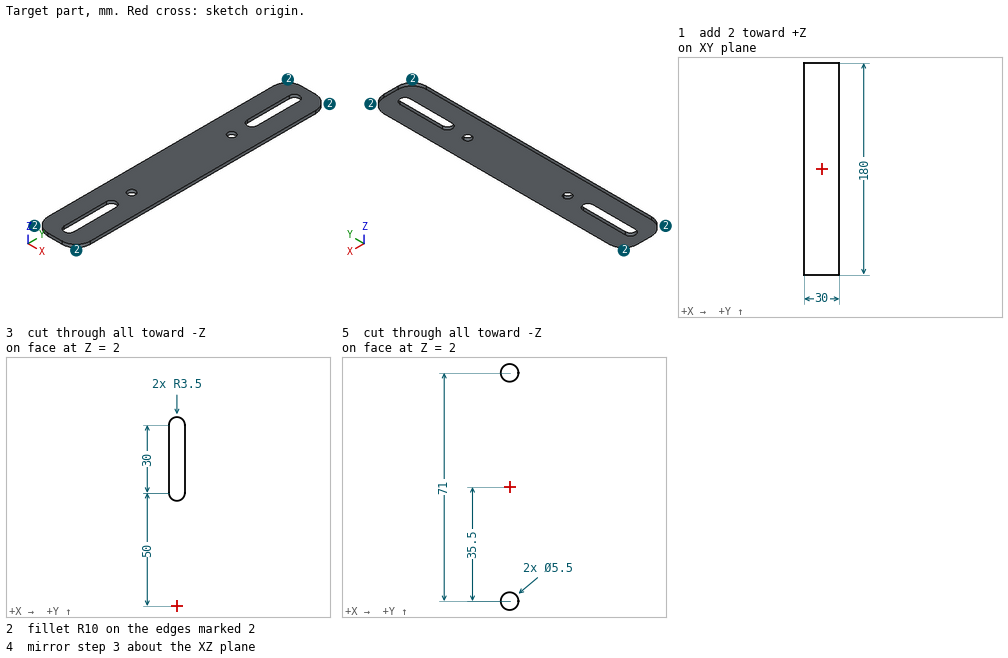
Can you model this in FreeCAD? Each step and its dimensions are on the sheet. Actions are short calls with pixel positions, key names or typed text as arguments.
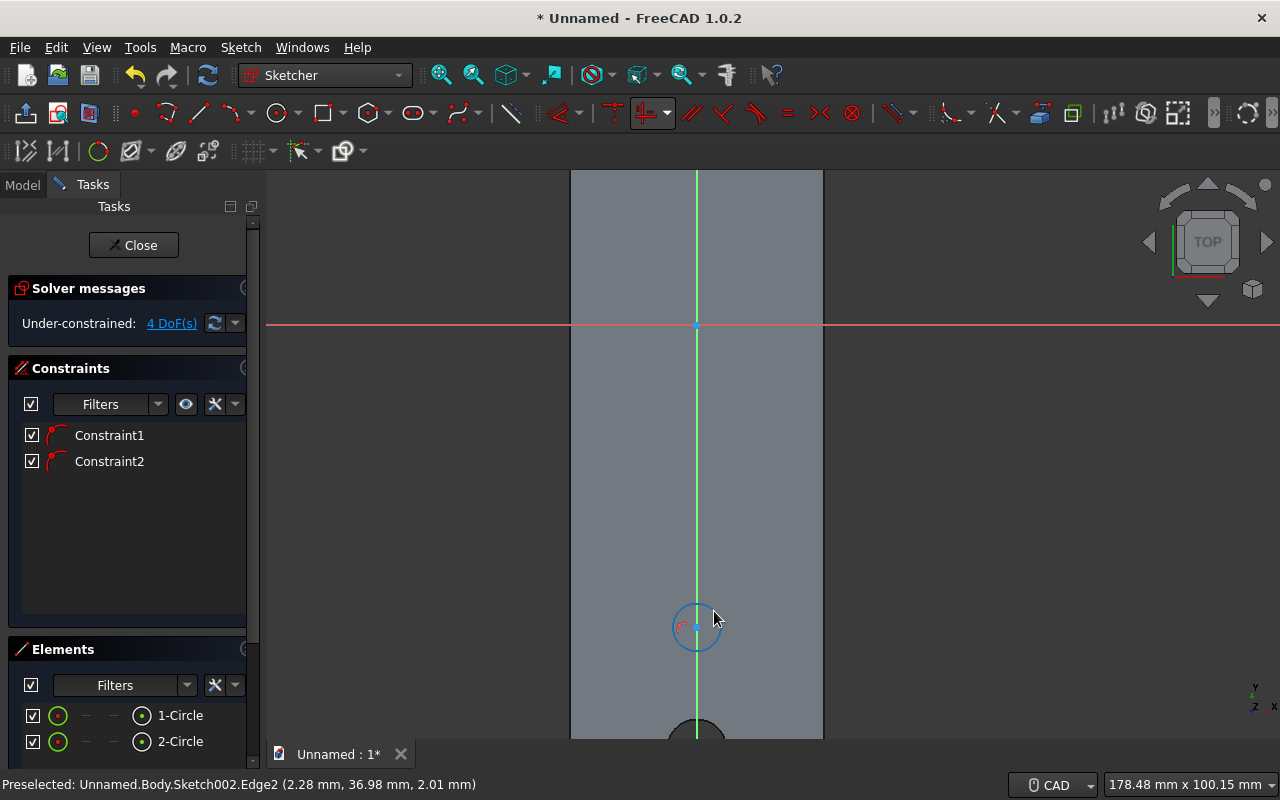
click(714, 610)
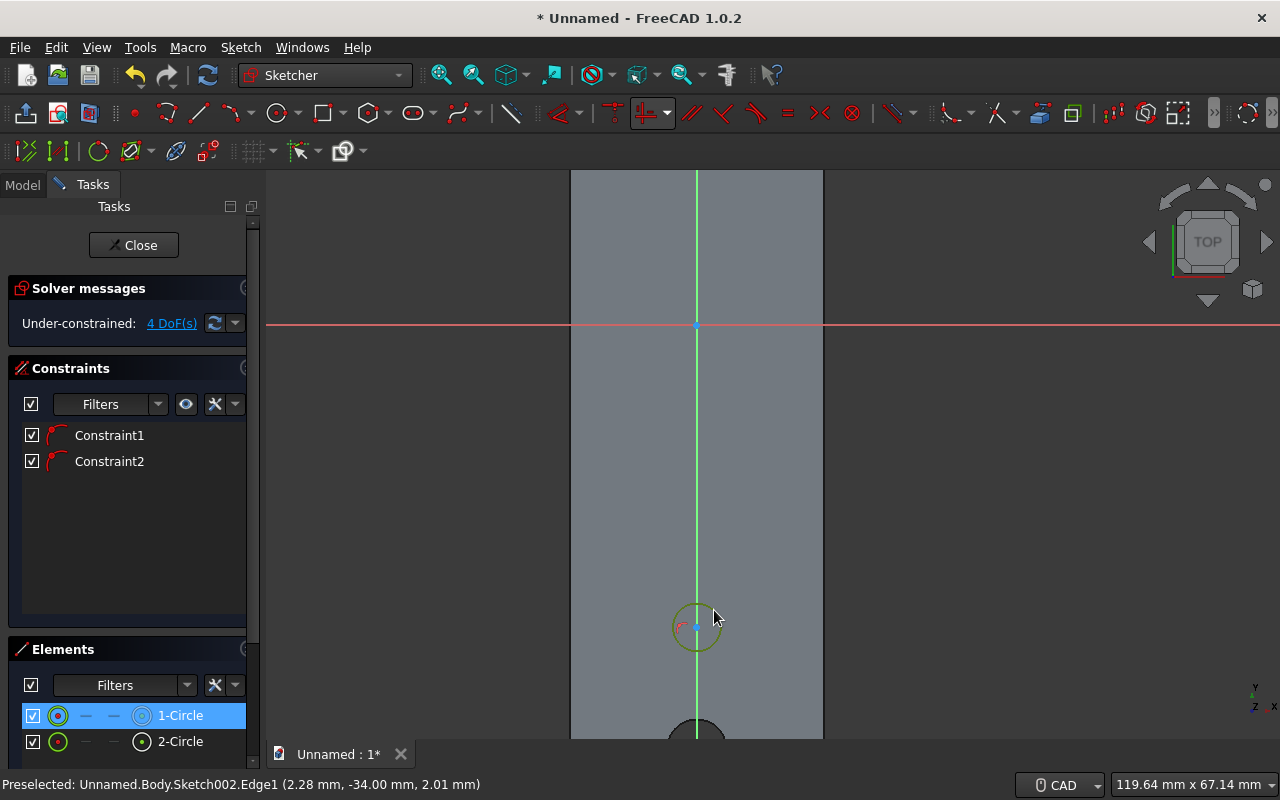
scroll(714, 612, down, 3)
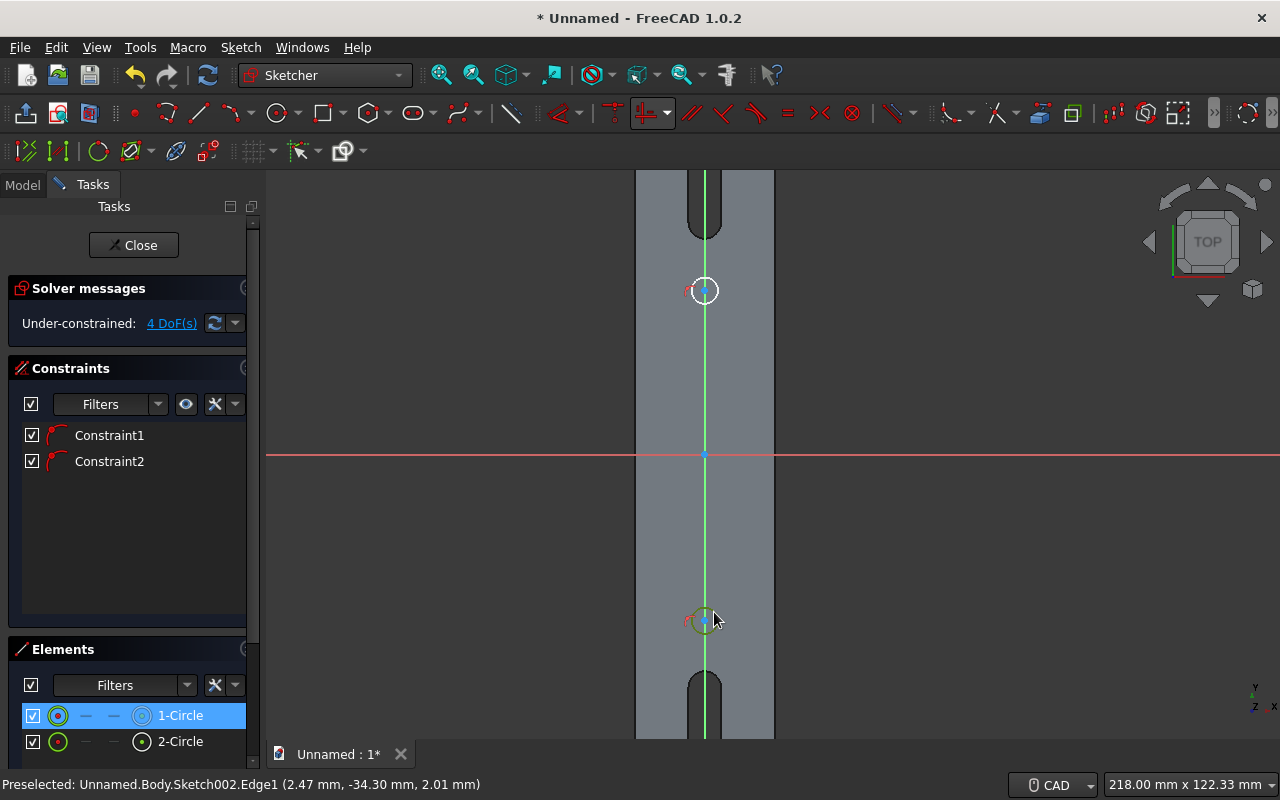
scroll(714, 281, up, 3)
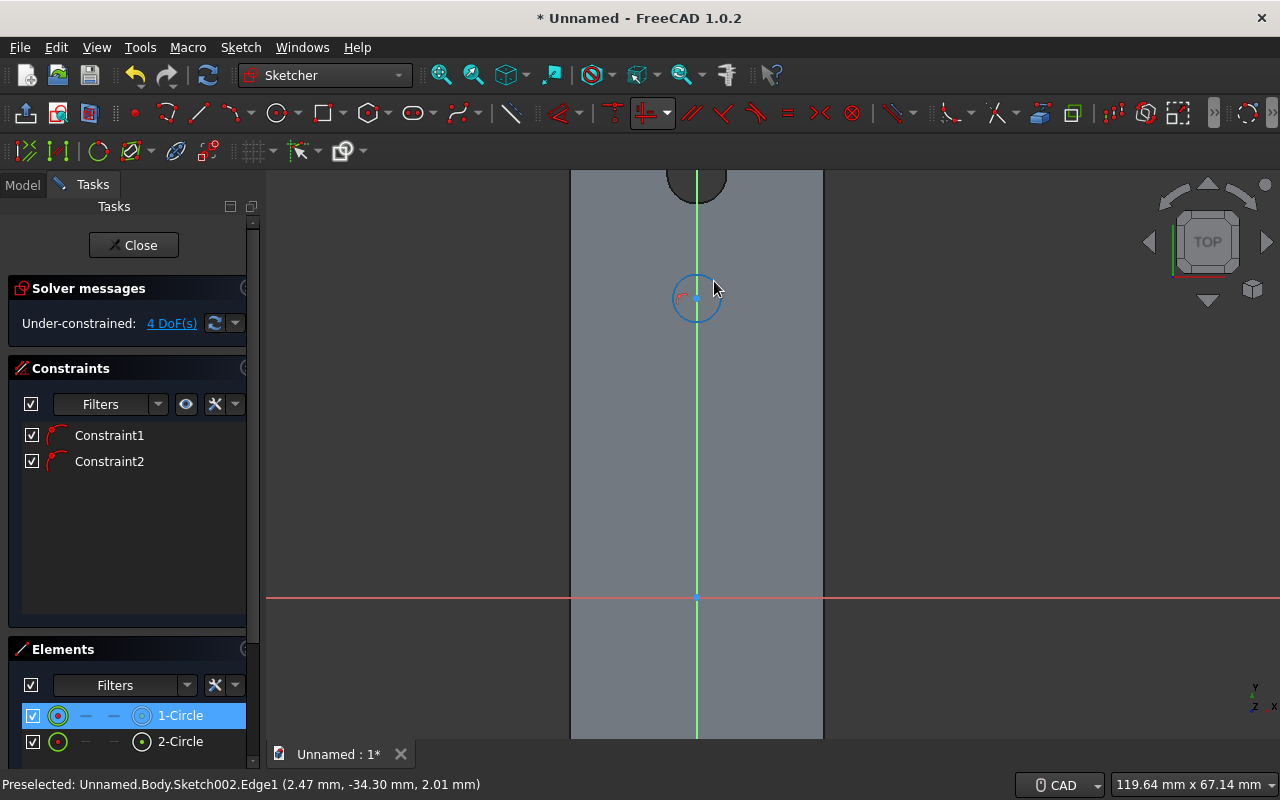
click(714, 281)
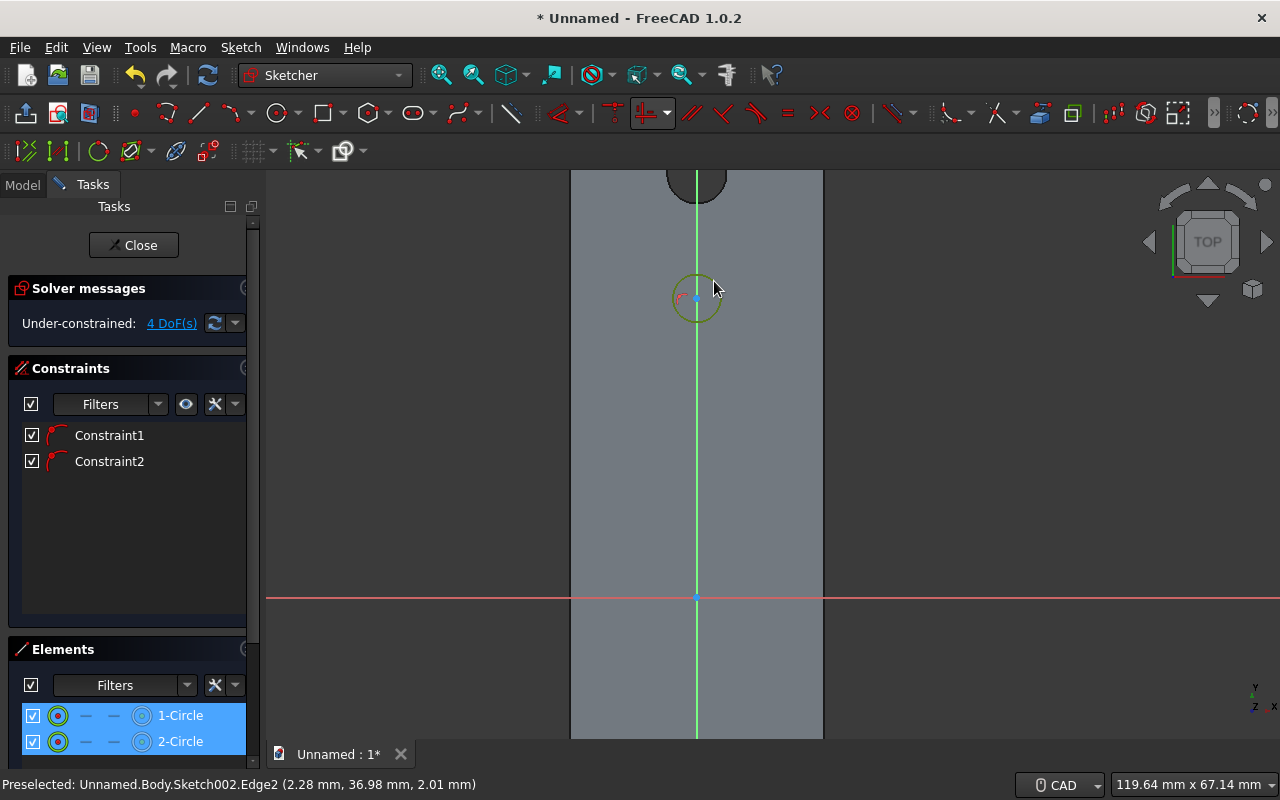
key(e)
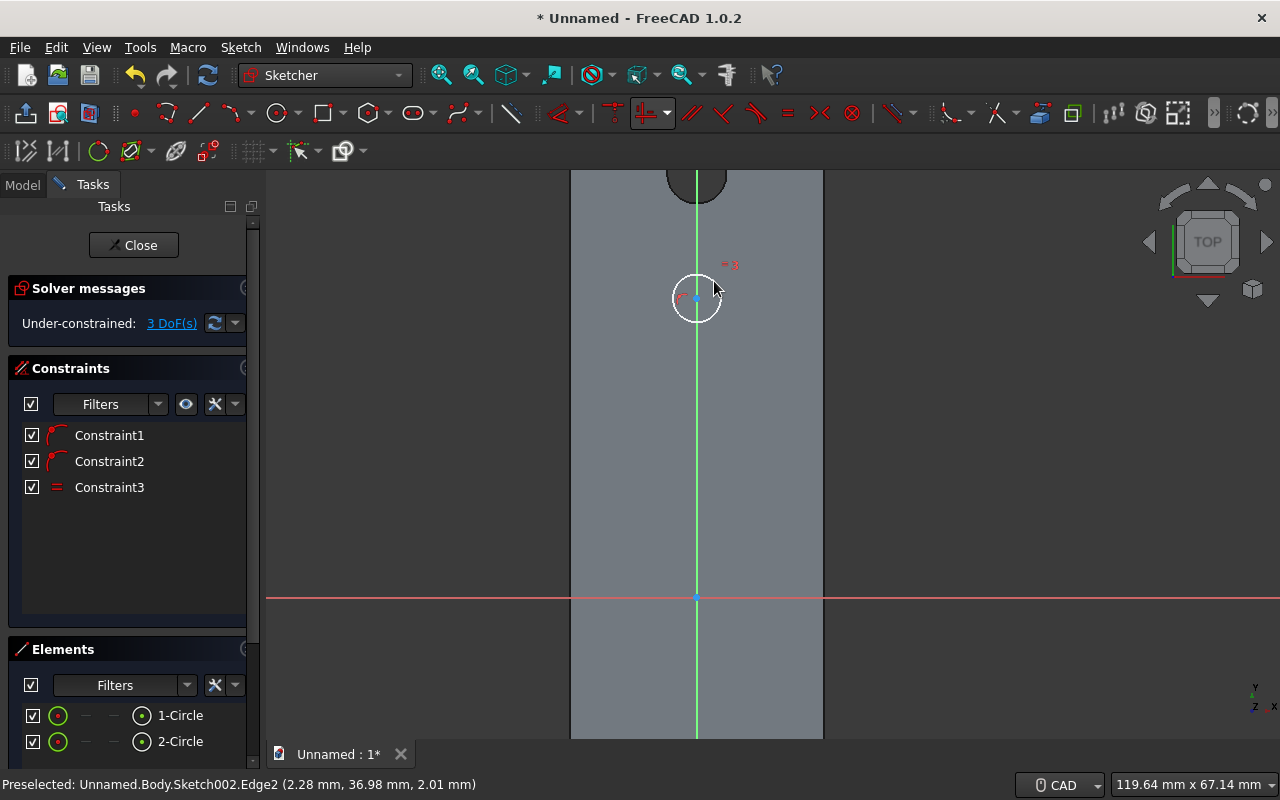
key(d)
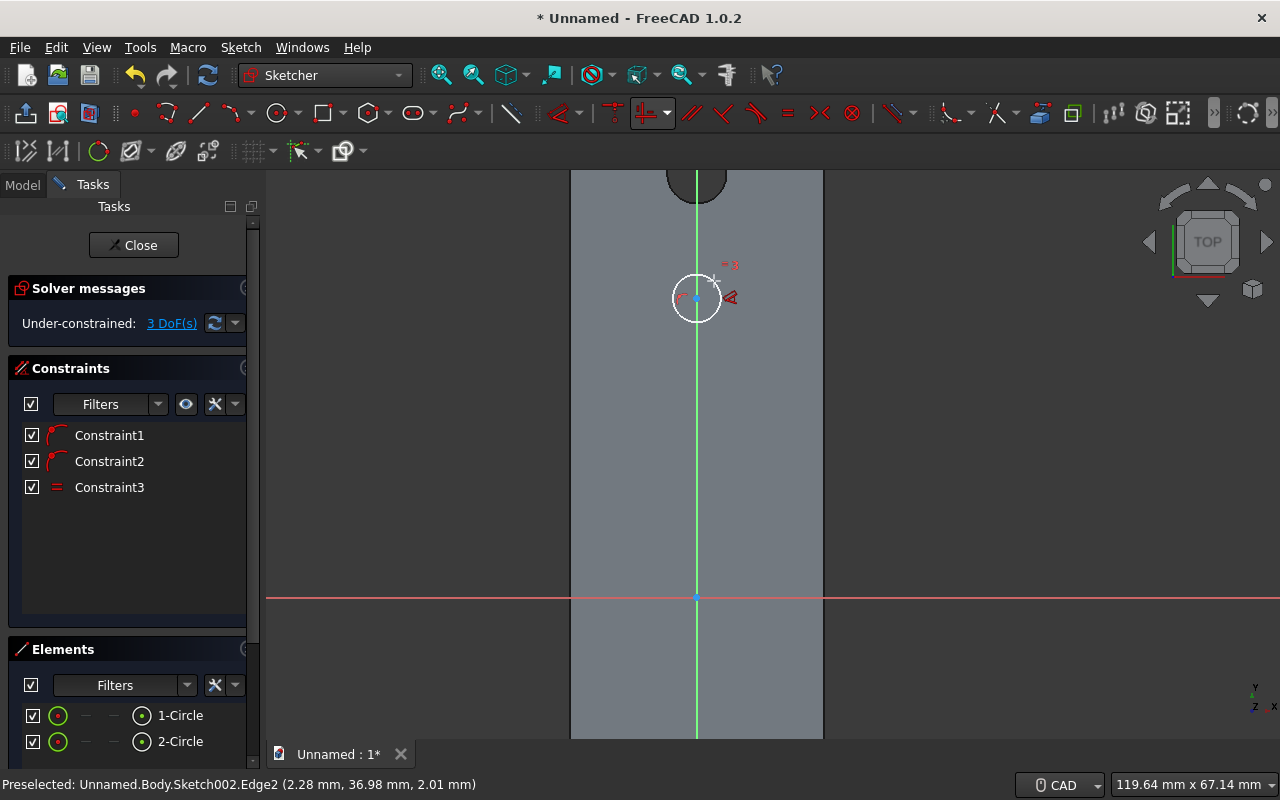
scroll(714, 280, down, 3)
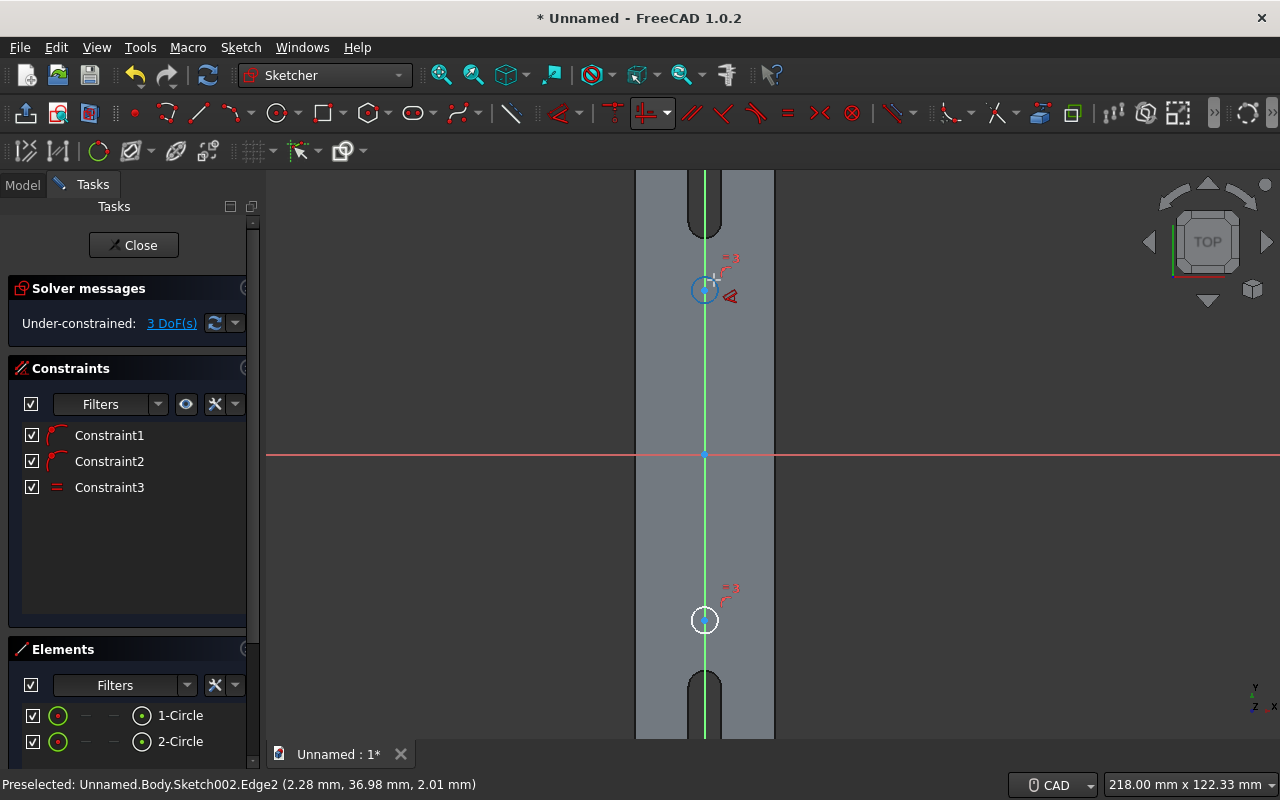
scroll(714, 611, up, 3)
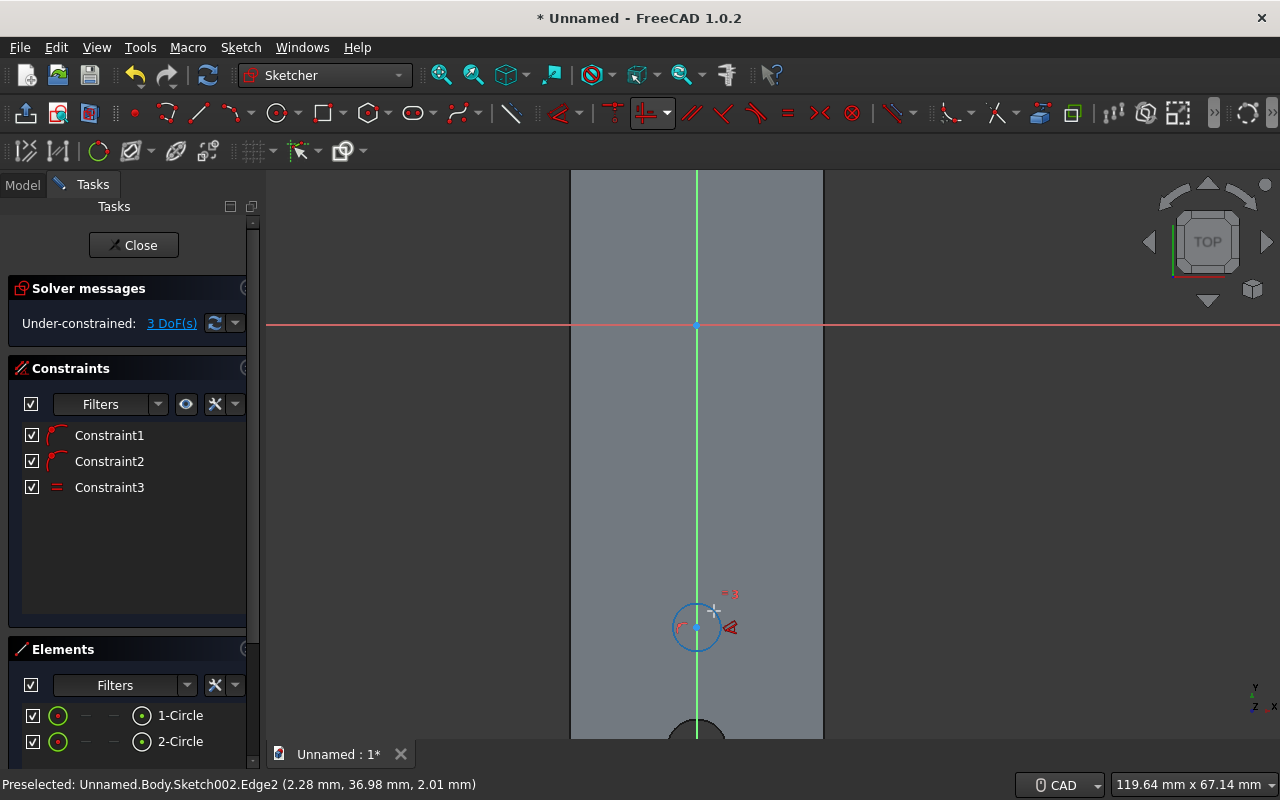
click(714, 610)
click(736, 587)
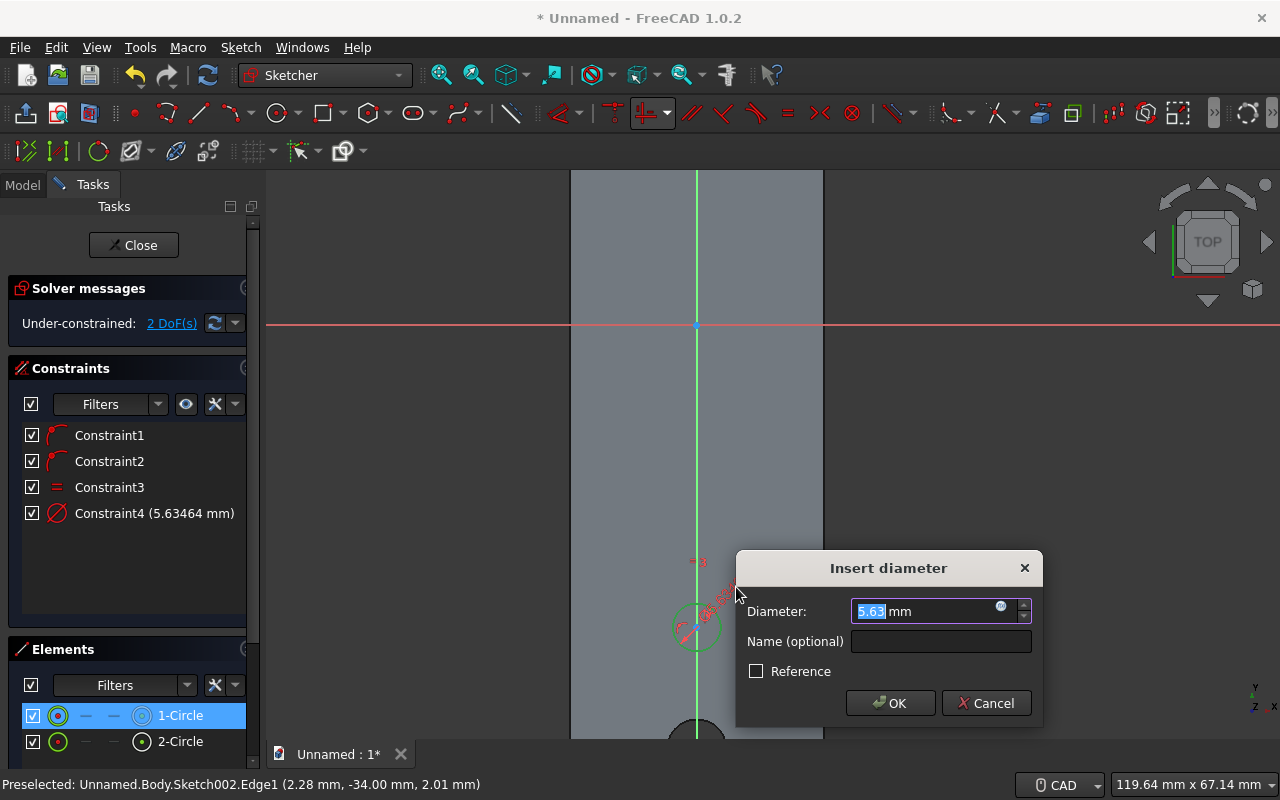
text(5.5)
key(Return)